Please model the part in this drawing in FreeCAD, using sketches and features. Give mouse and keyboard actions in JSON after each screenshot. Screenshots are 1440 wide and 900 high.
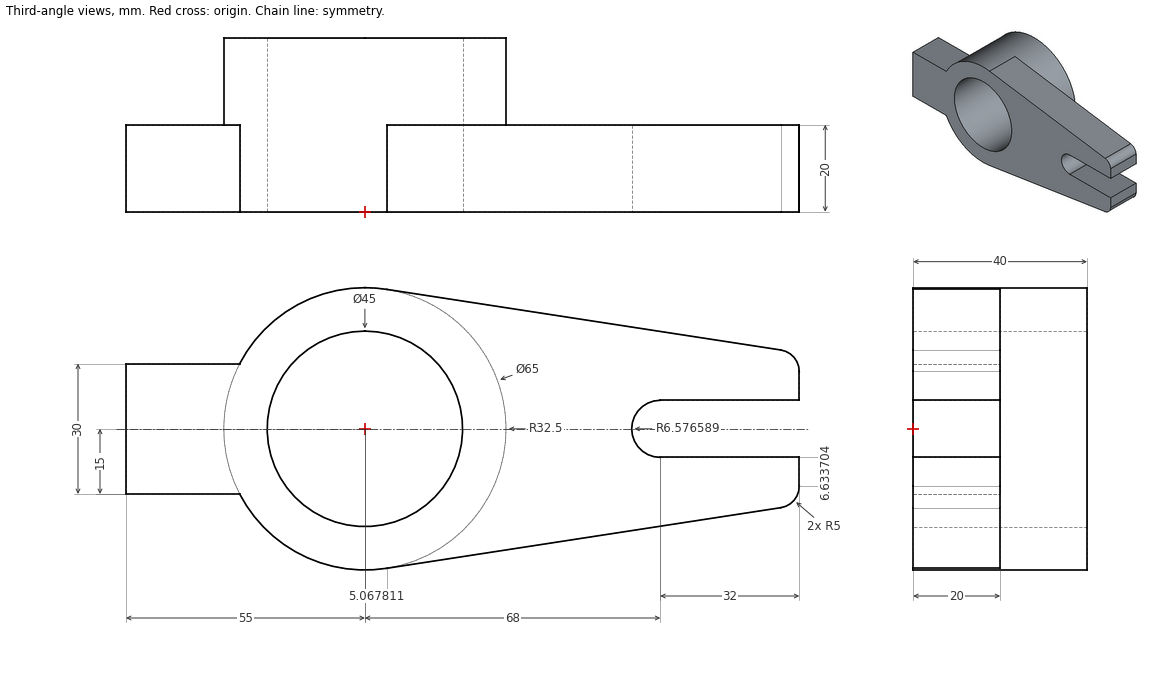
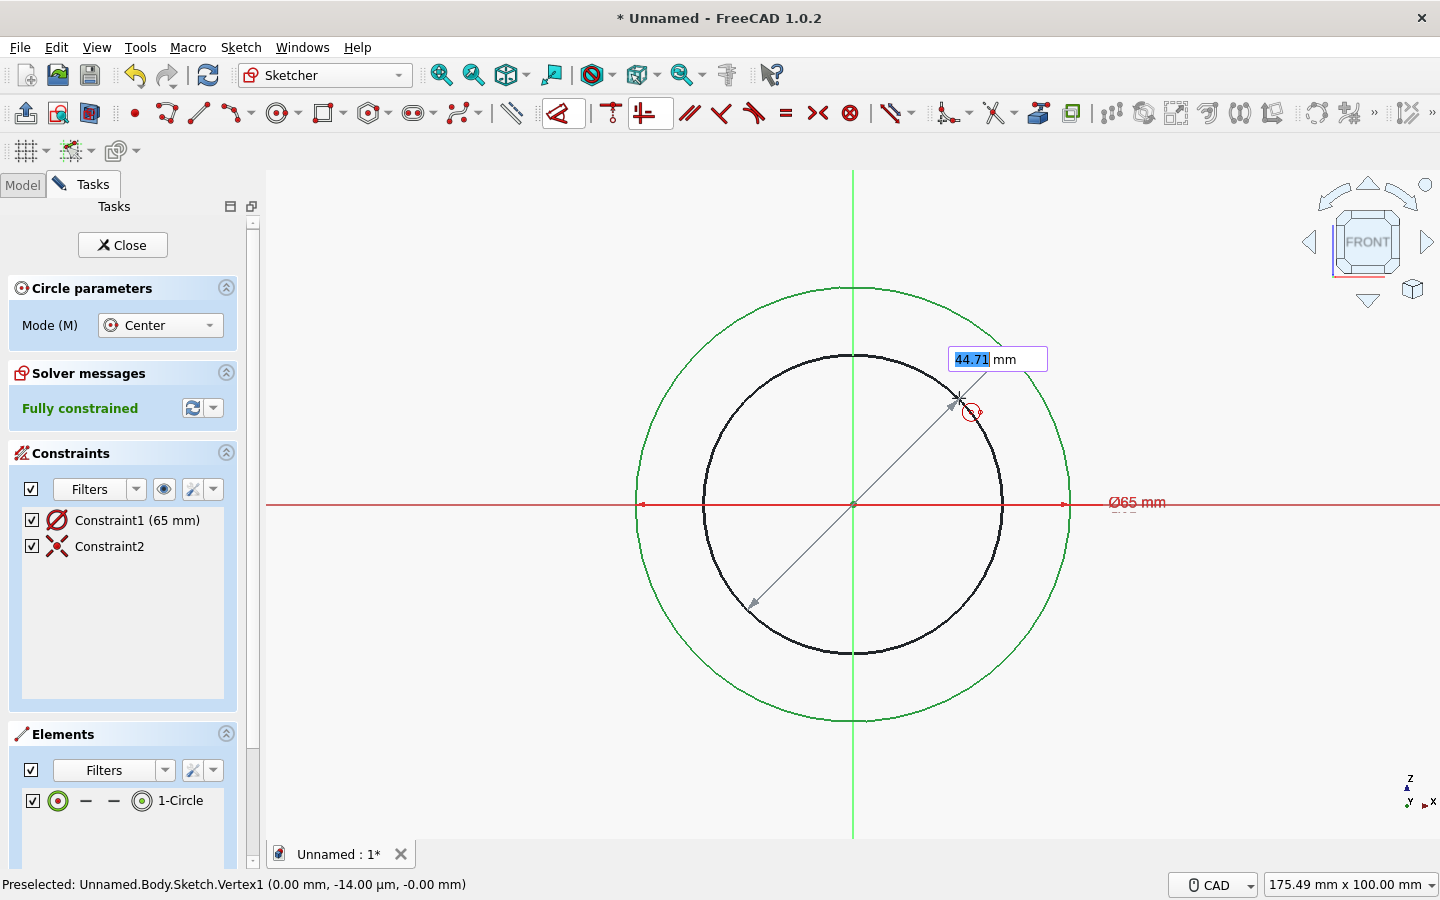
{"action": "type", "text": "45"}
{"action": "key", "text": "Return"}
{"action": "key", "text": "Escape"}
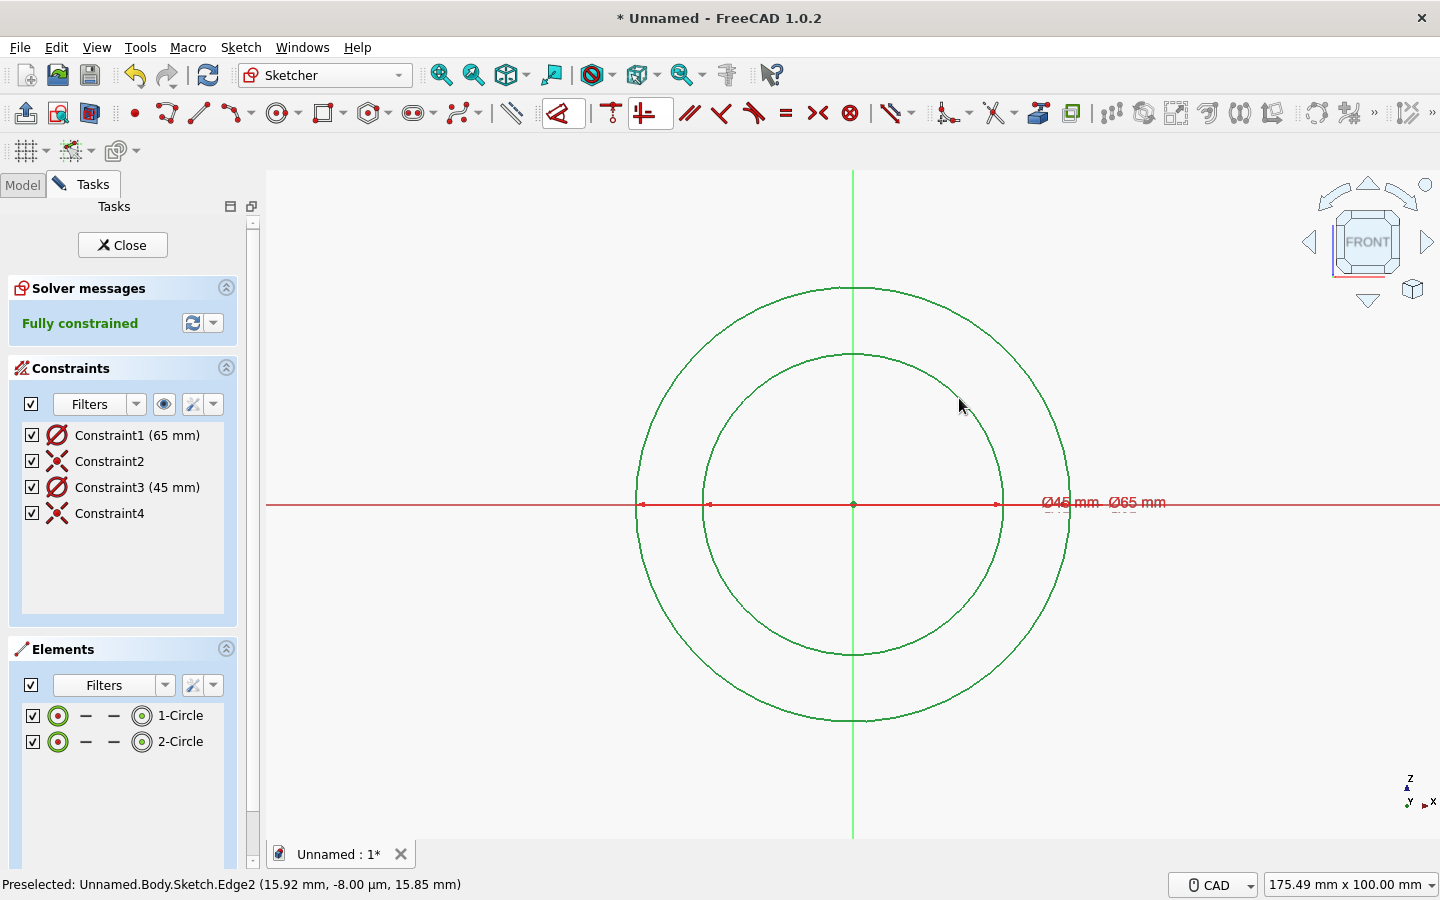
{"action": "left_click", "coordinate": [123, 245]}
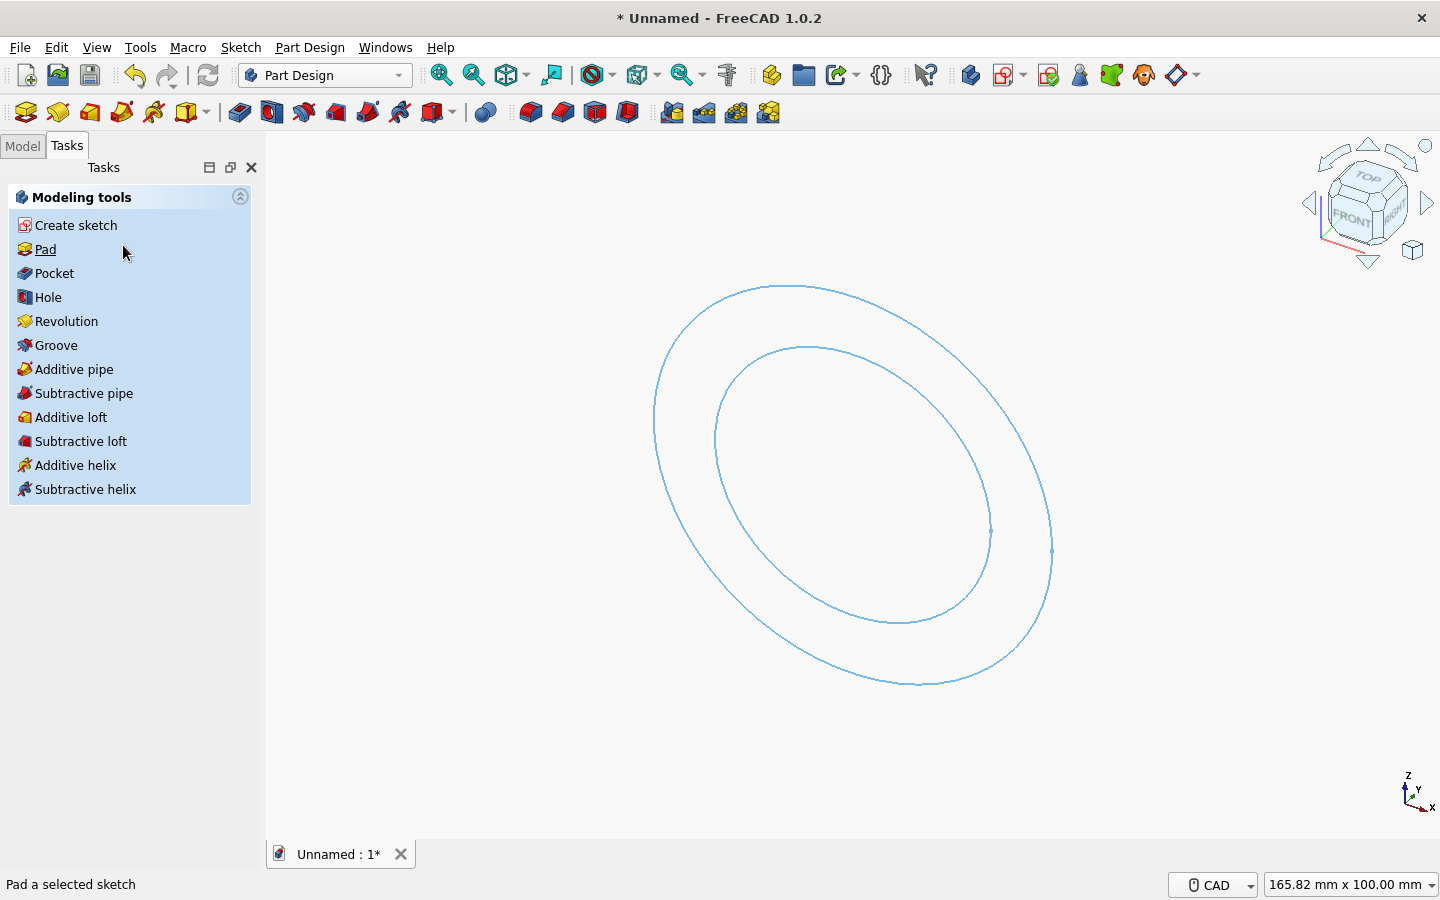
{"action": "left_click", "coordinate": [26, 112]}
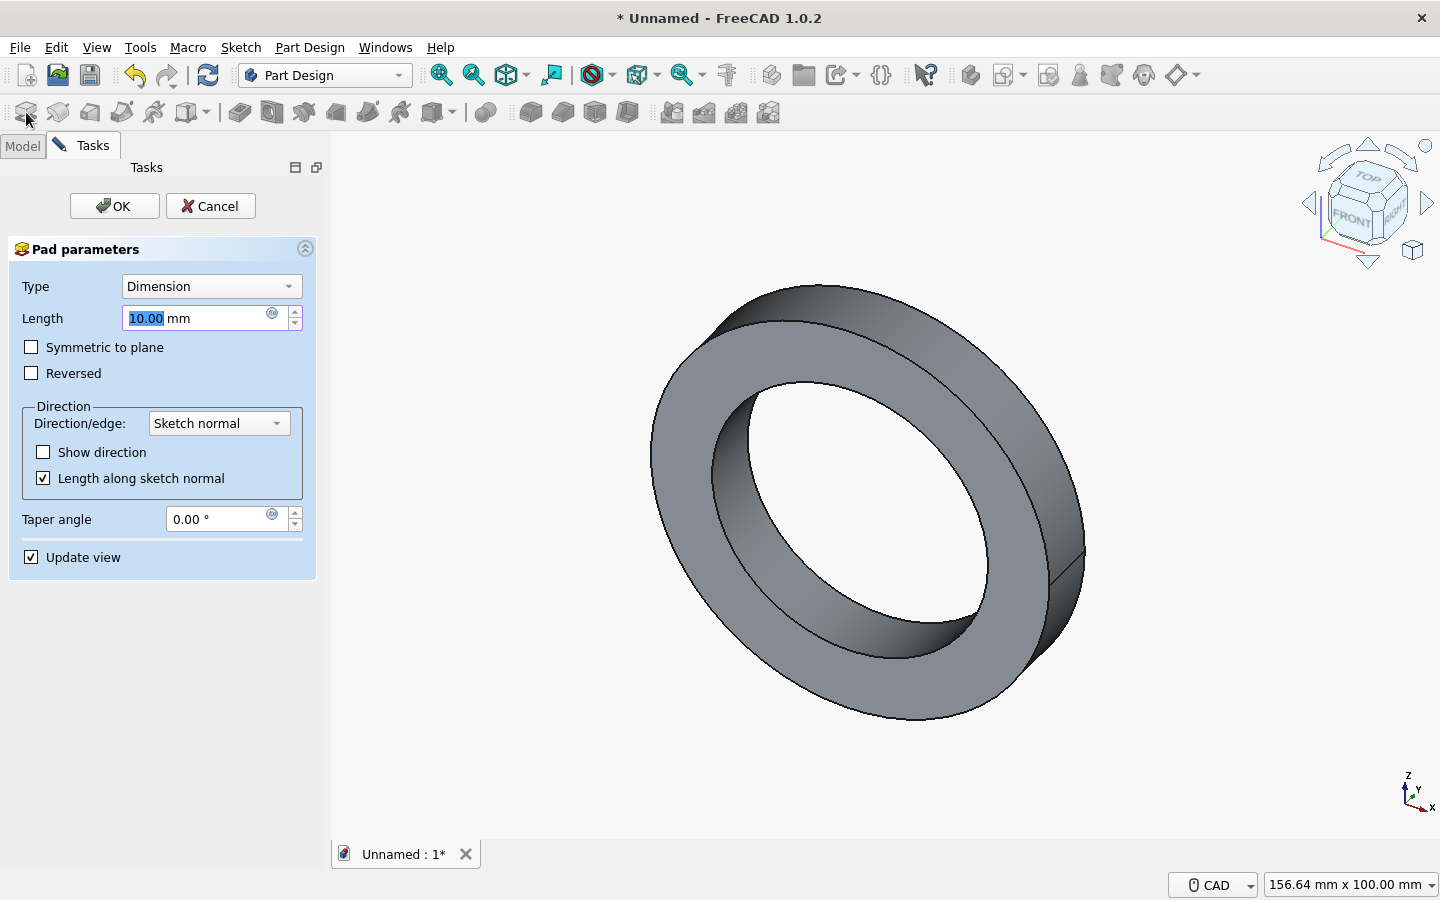
{"action": "type", "text": "40"}
{"action": "key", "text": "Tab"}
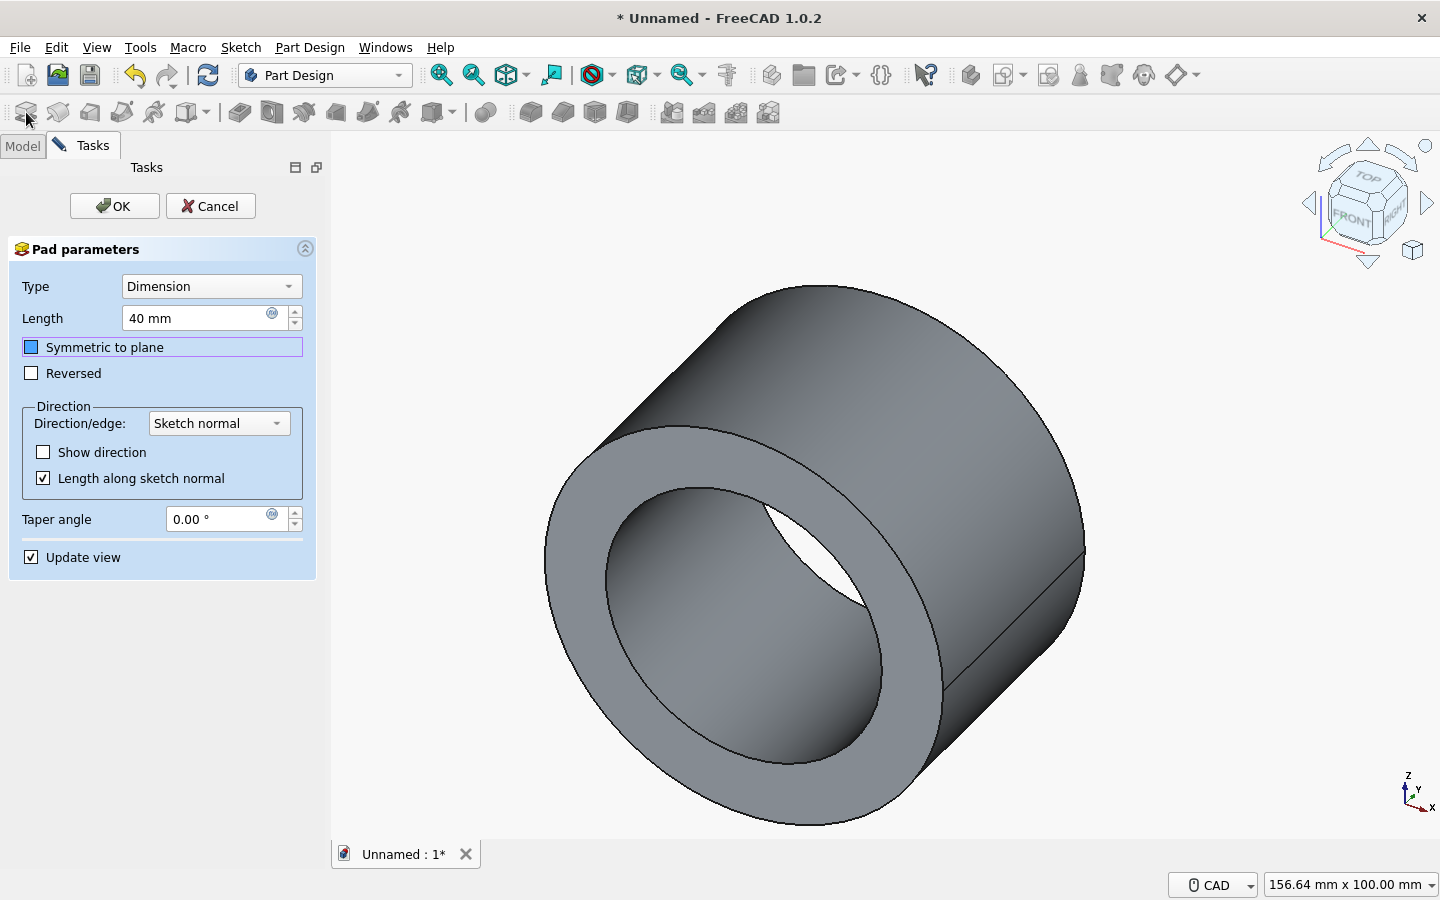
{"action": "left_click", "coordinate": [30, 373]}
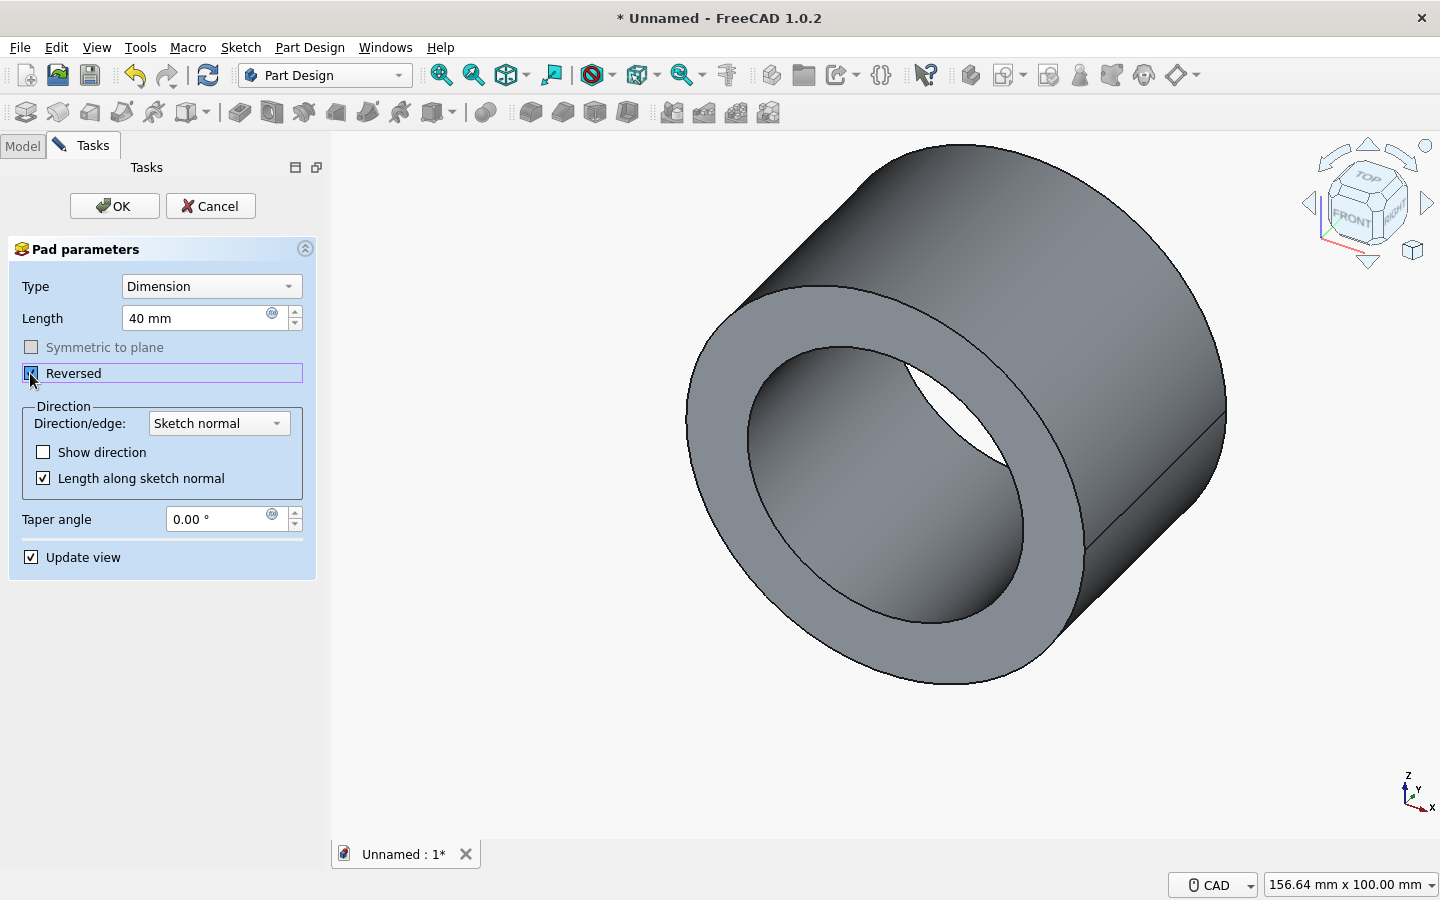
{"action": "left_click", "coordinate": [115, 206]}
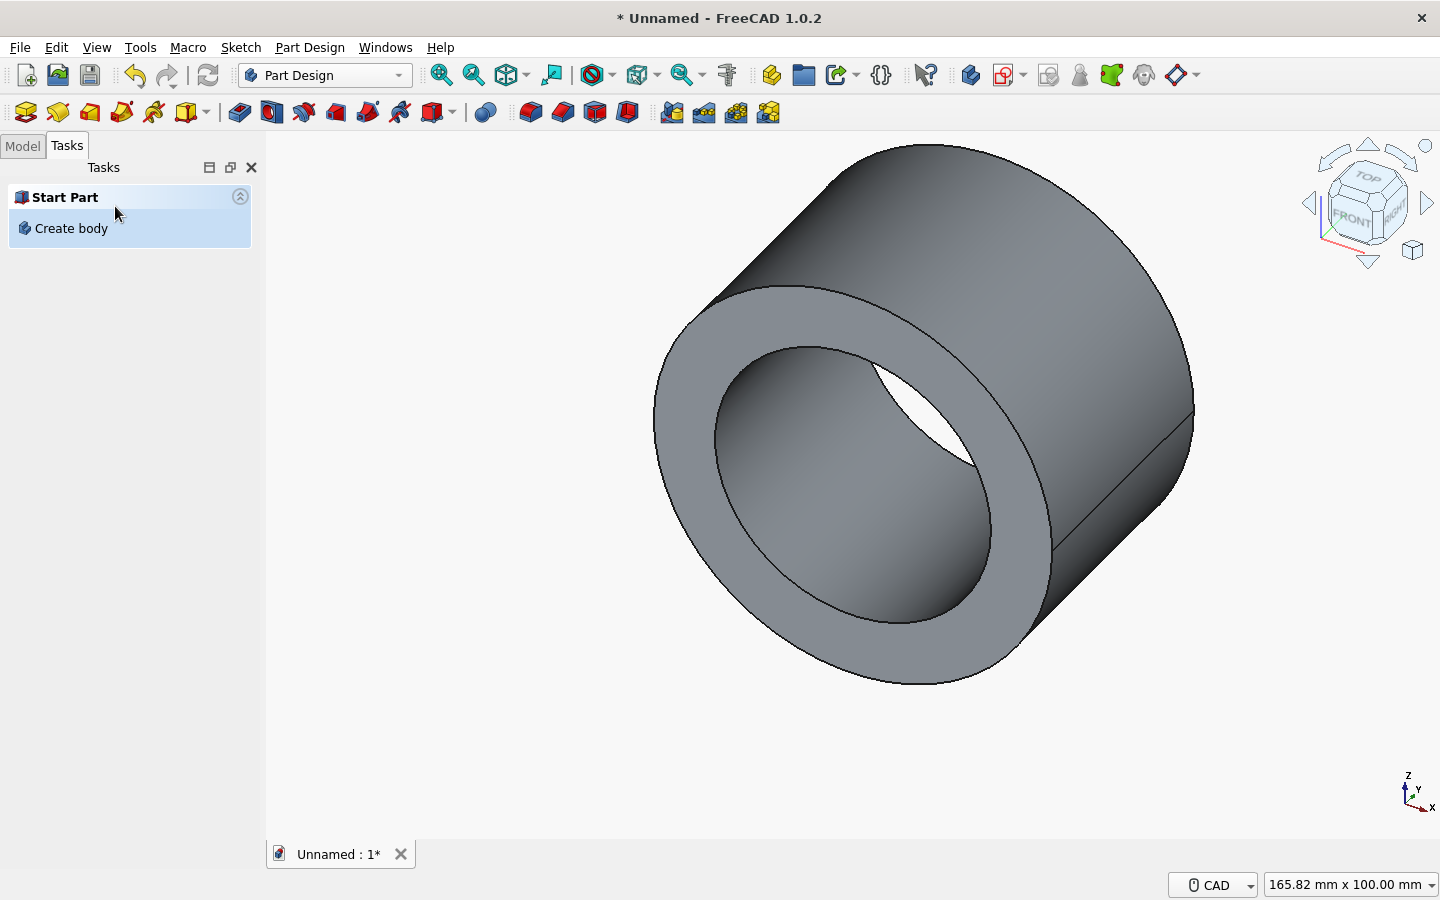
{"action": "left_click", "coordinate": [442, 76]}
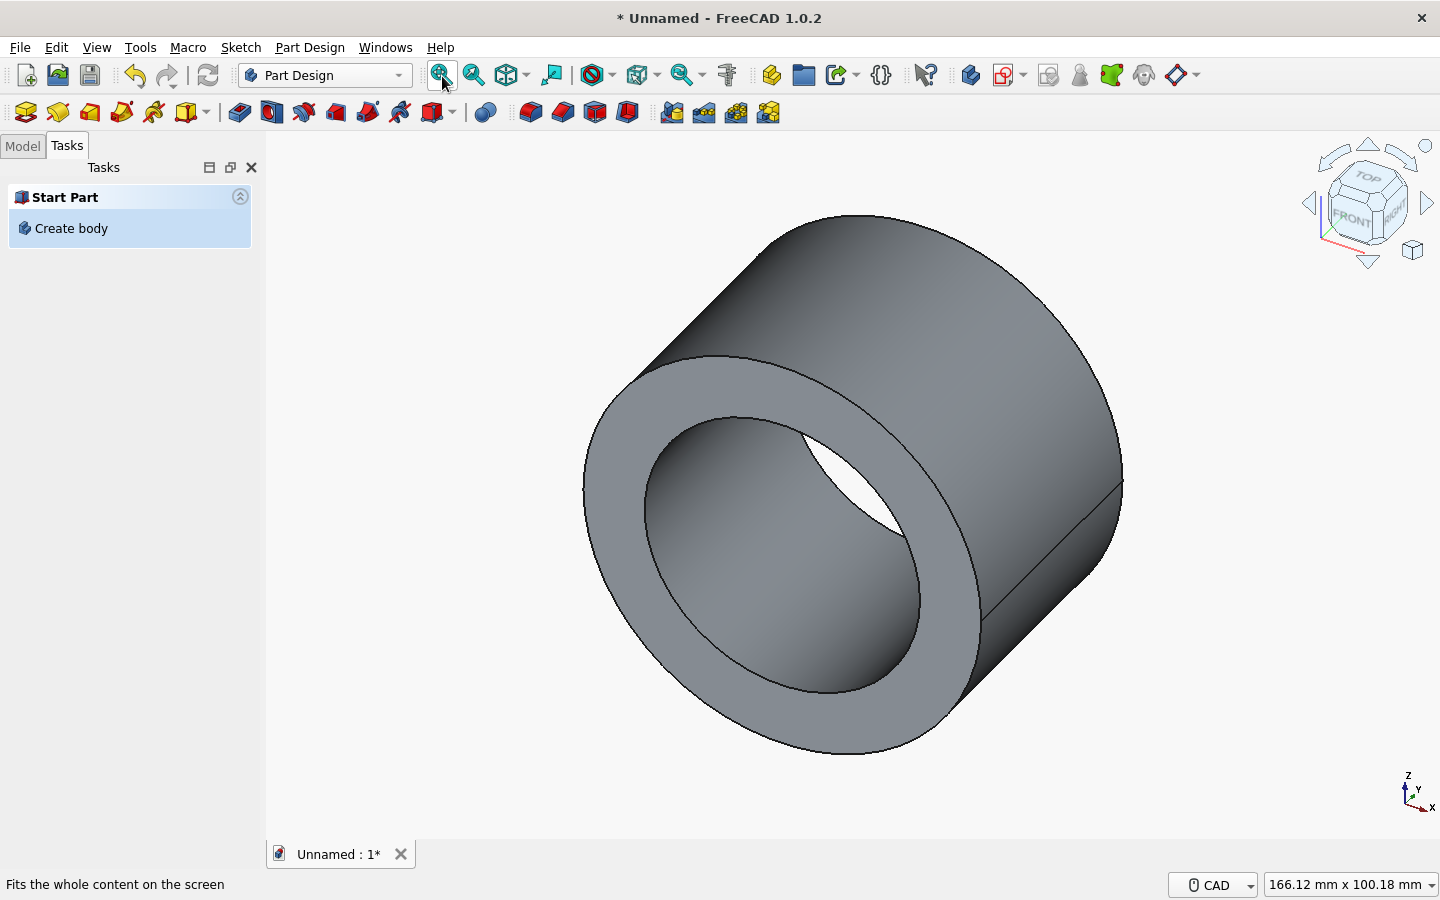
{"action": "left_click", "coordinate": [953, 611]}